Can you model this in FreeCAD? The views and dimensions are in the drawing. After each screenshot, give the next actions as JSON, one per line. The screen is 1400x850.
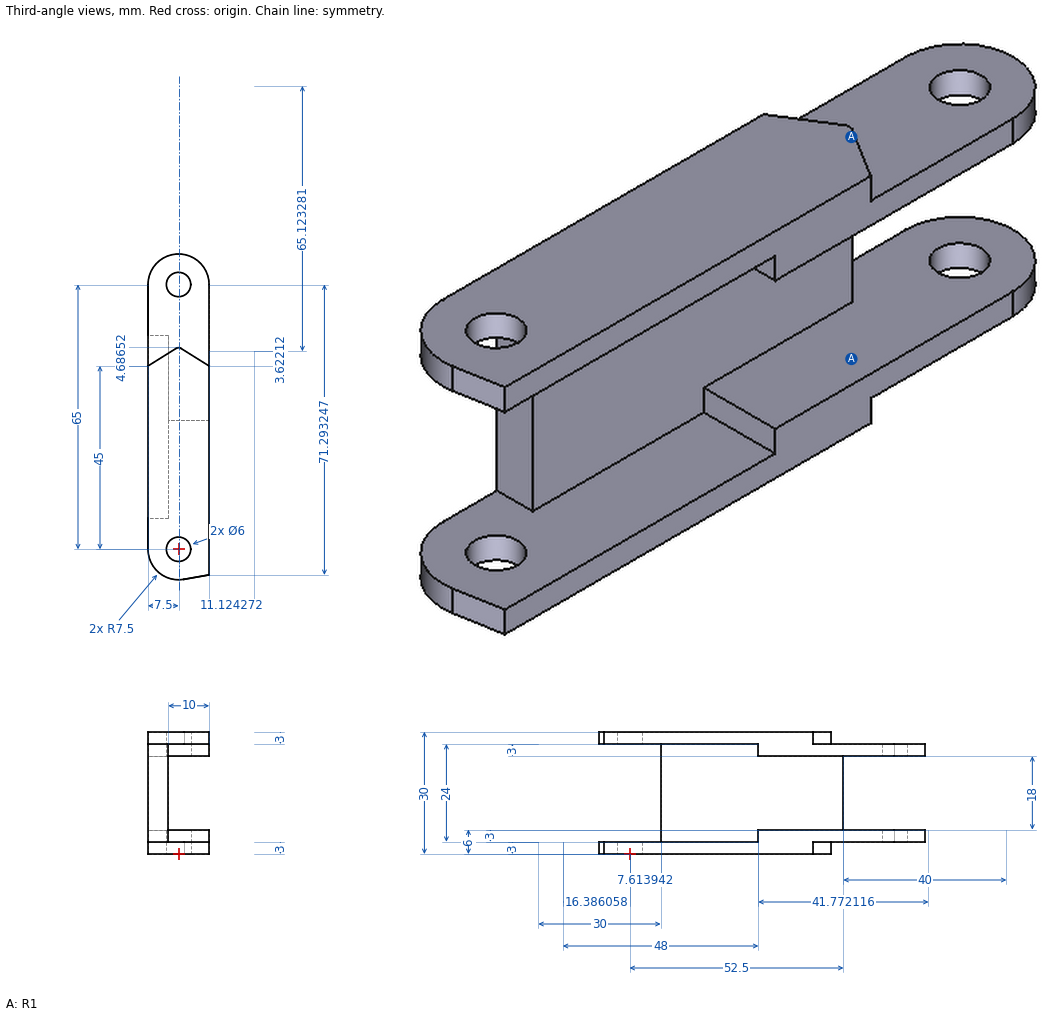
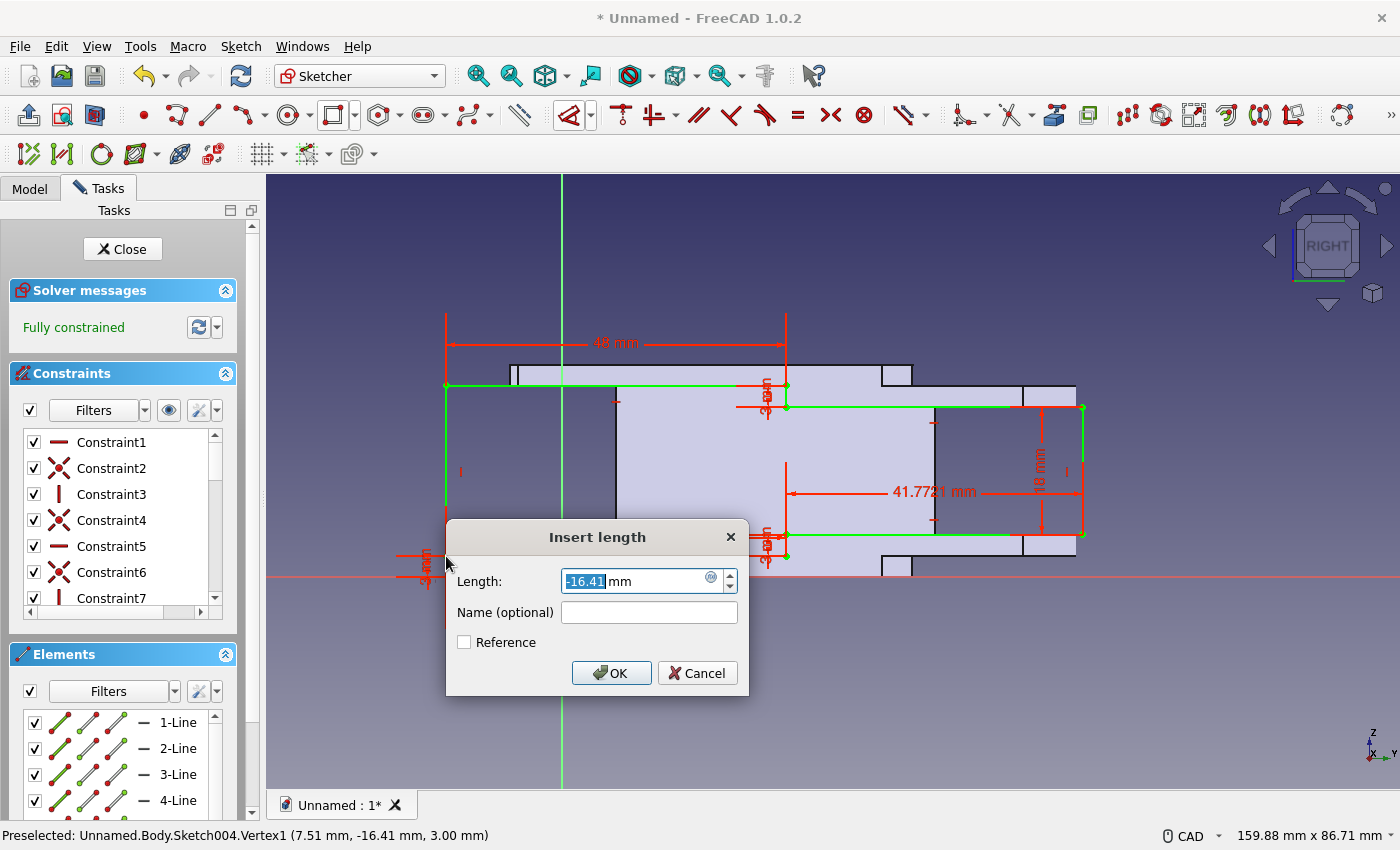
{"action": "type", "text": "-16.386058"}
{"action": "key", "text": "Return"}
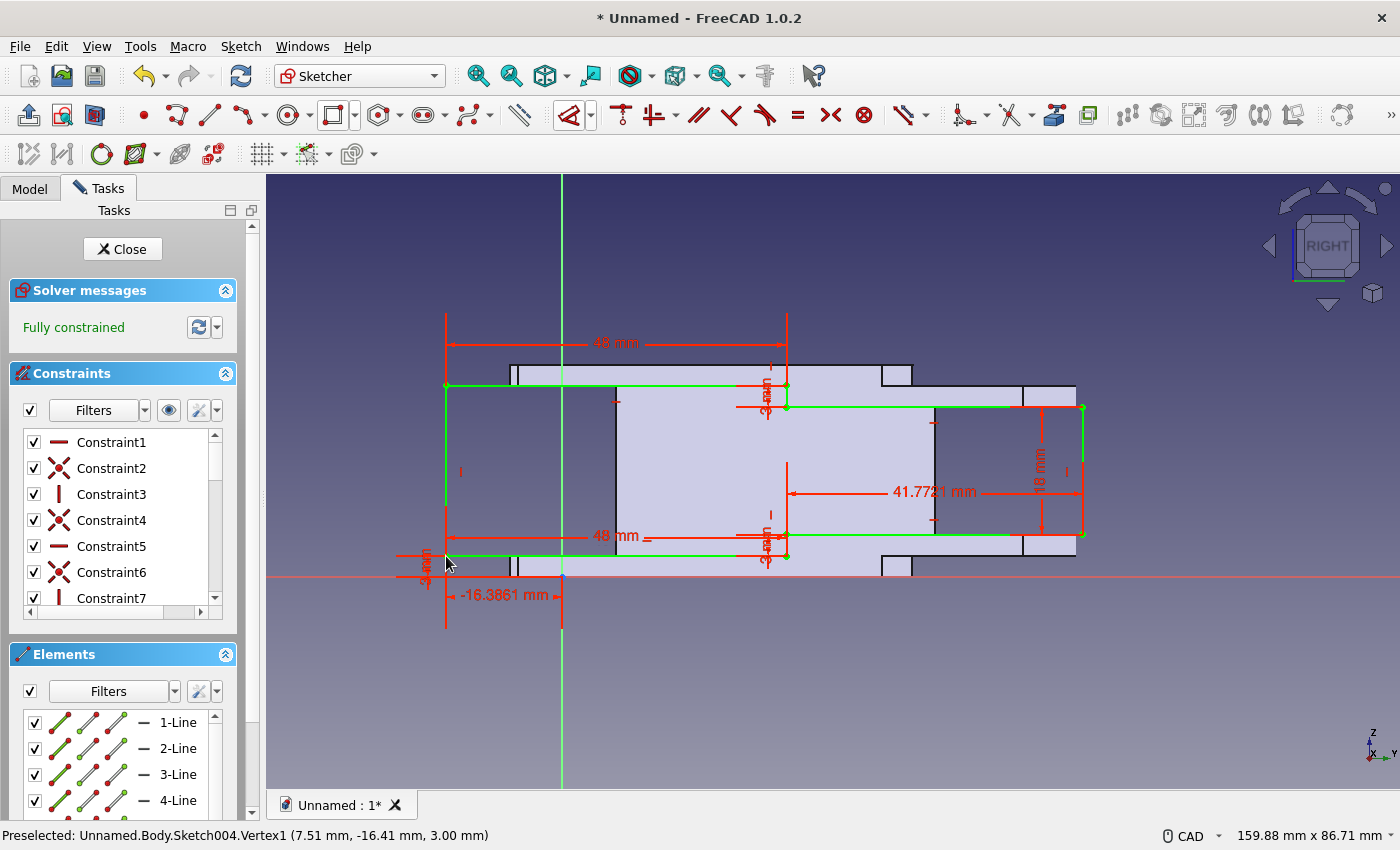
{"action": "left_click", "coordinate": [123, 249]}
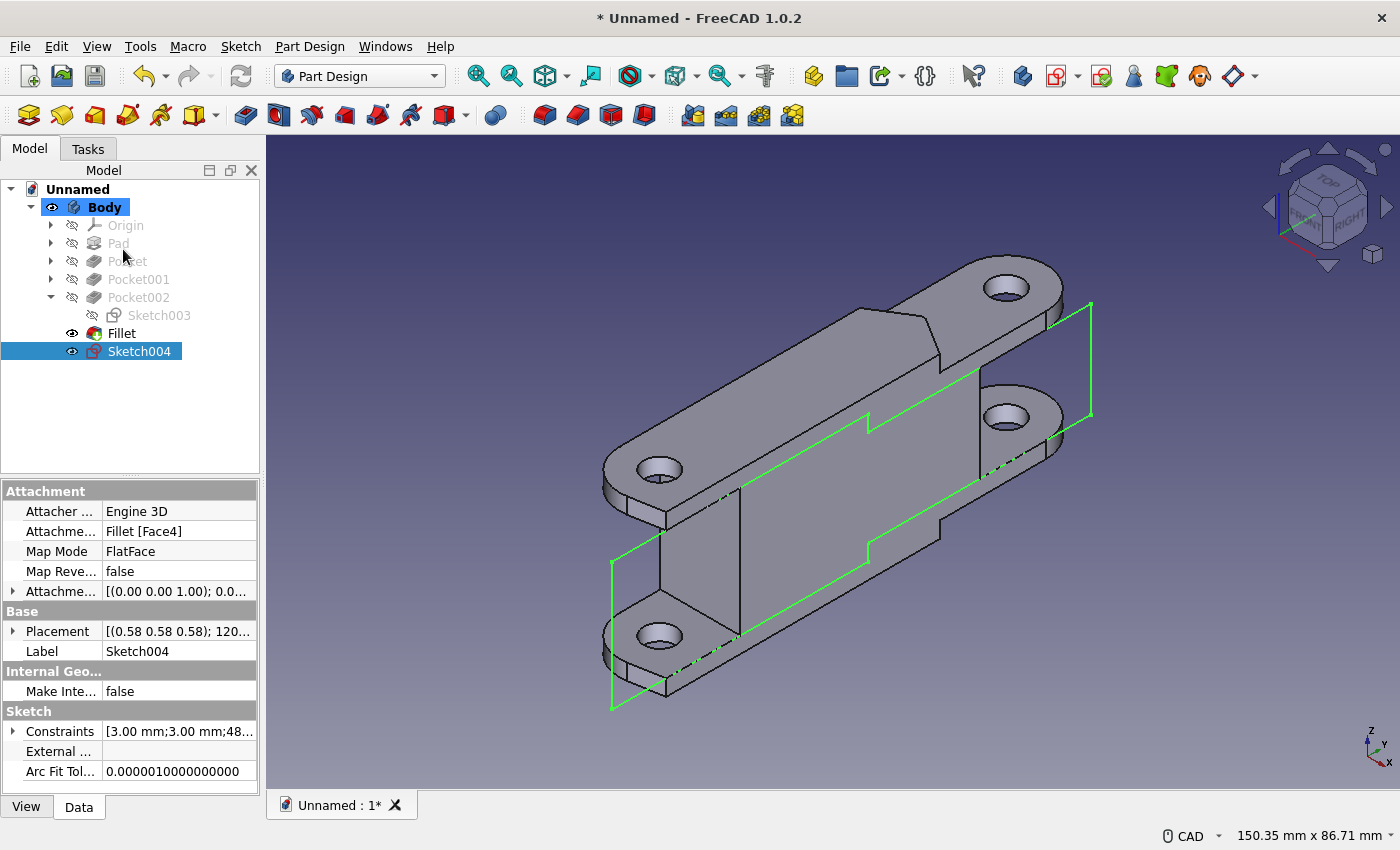
{"action": "left_click", "coordinate": [246, 116]}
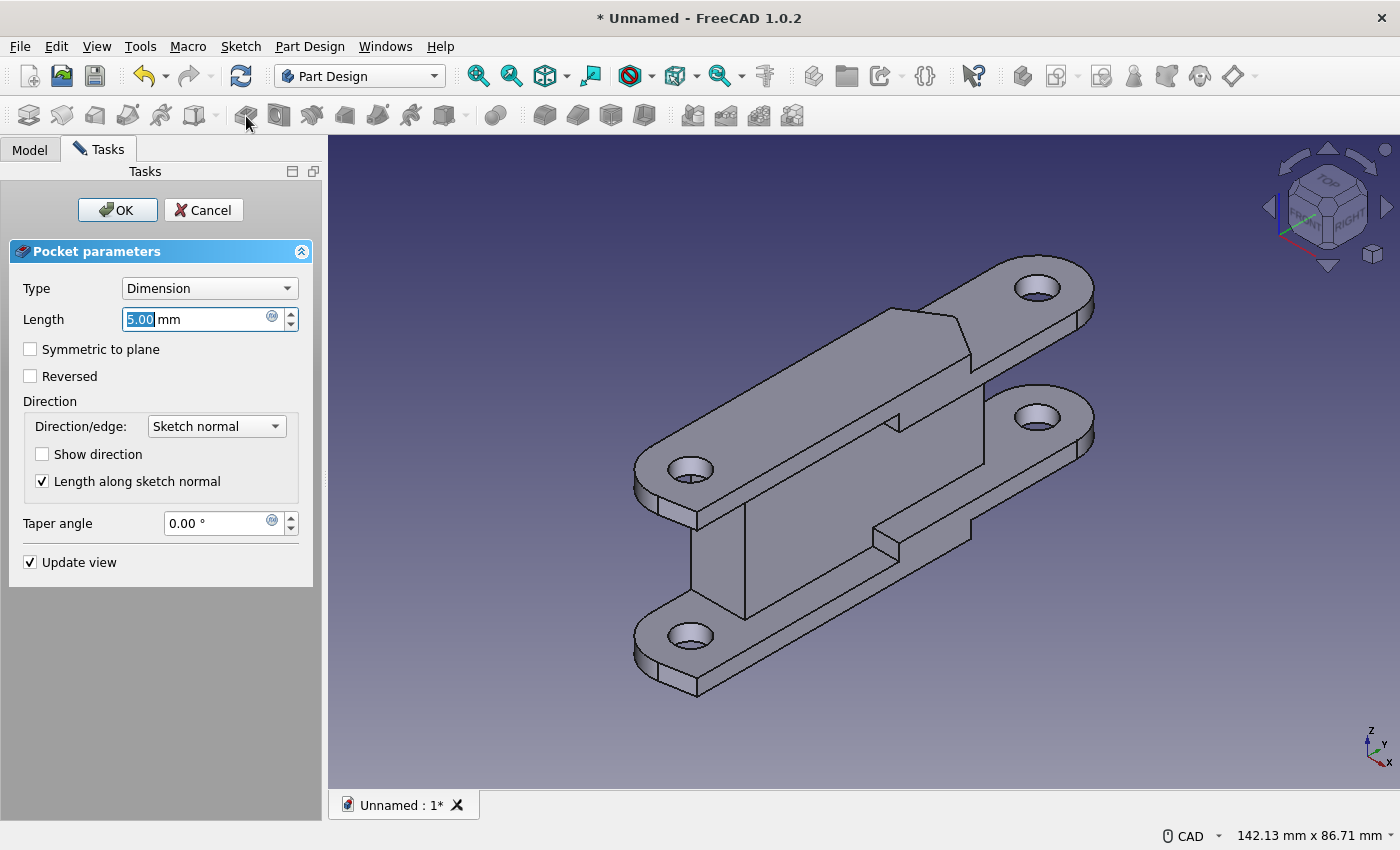
{"action": "type", "text": "10"}
{"action": "key", "text": "Tab"}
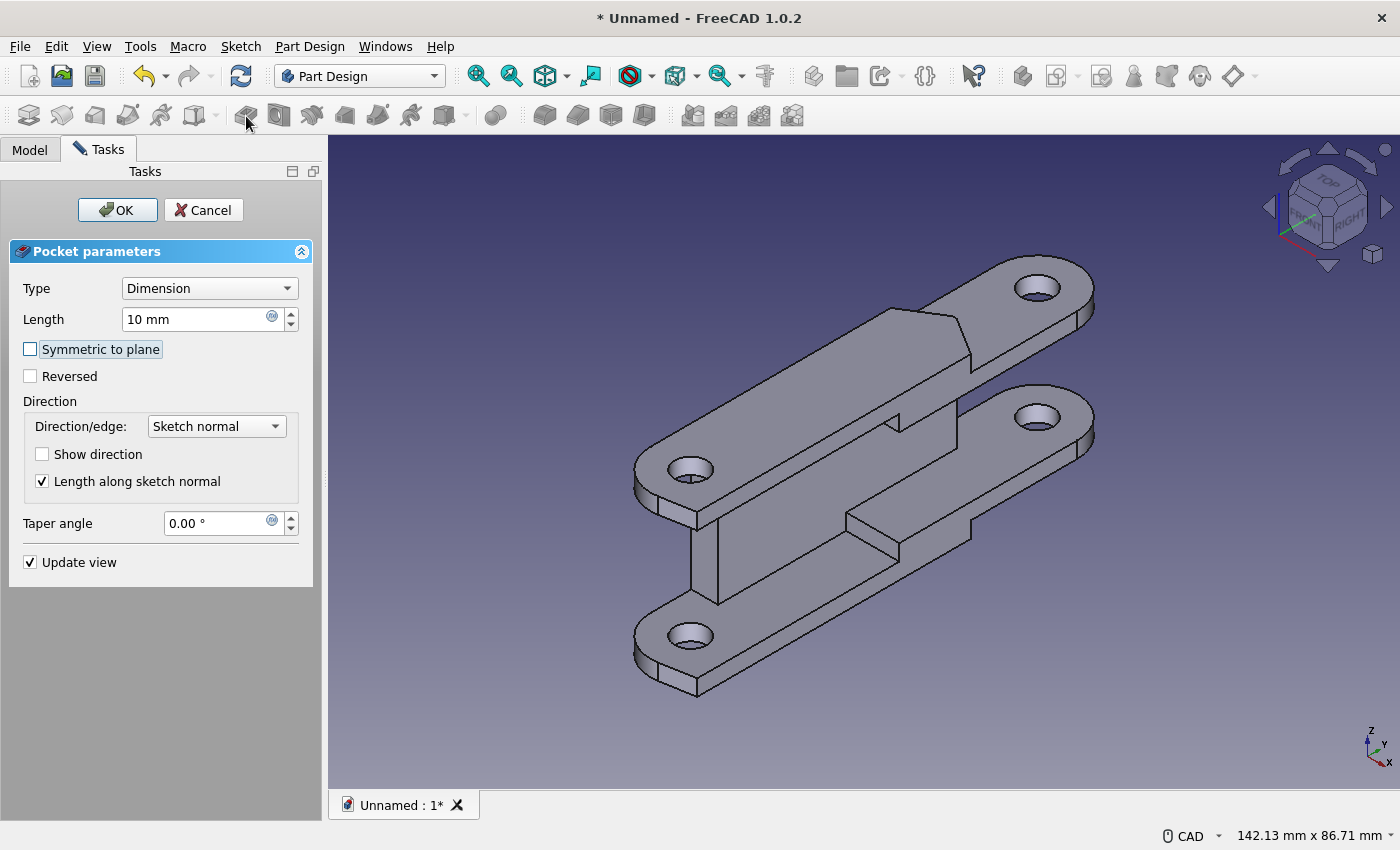
{"action": "left_click", "coordinate": [118, 210]}